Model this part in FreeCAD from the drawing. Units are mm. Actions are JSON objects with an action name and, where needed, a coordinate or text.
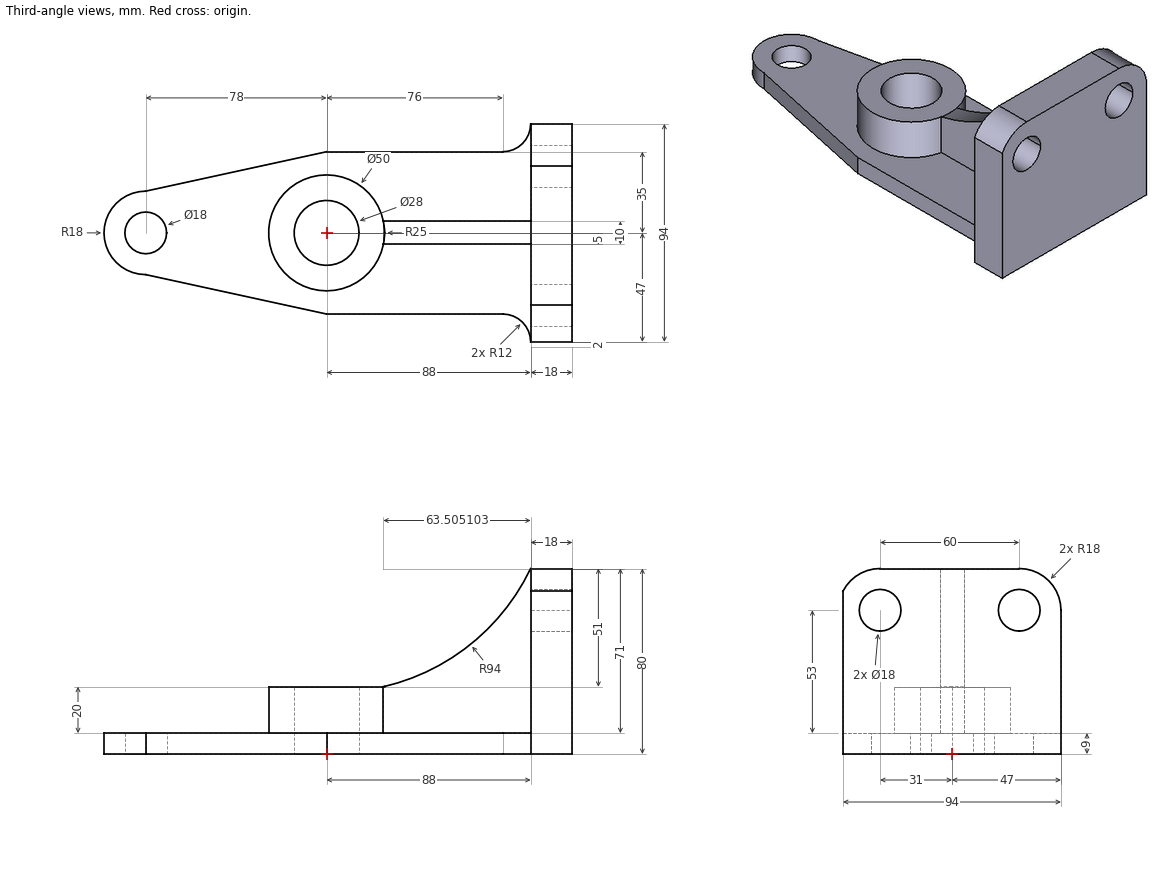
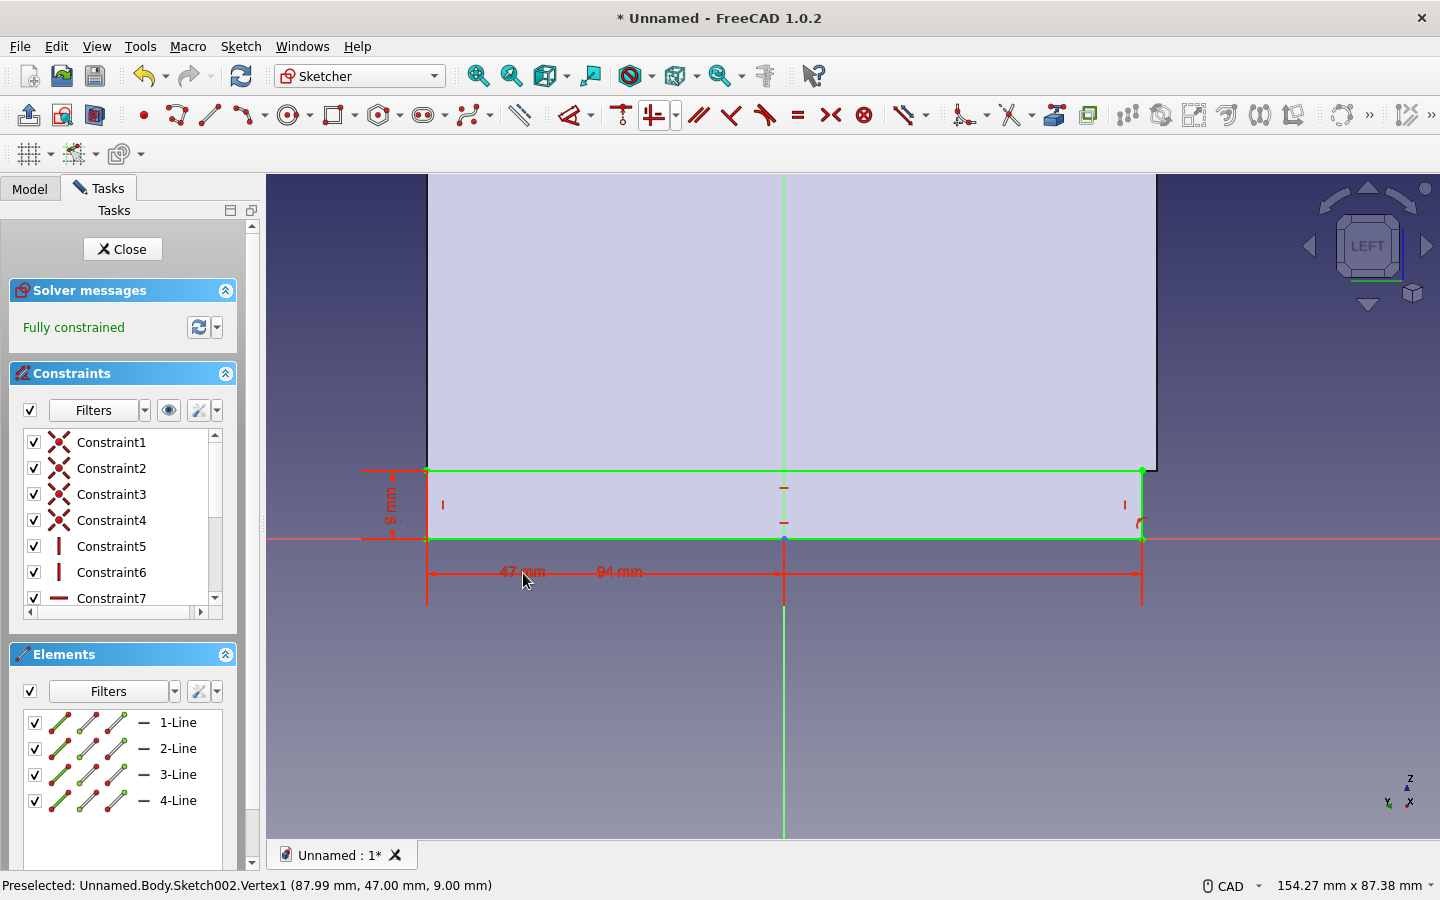
{"action": "left_click", "coordinate": [123, 249]}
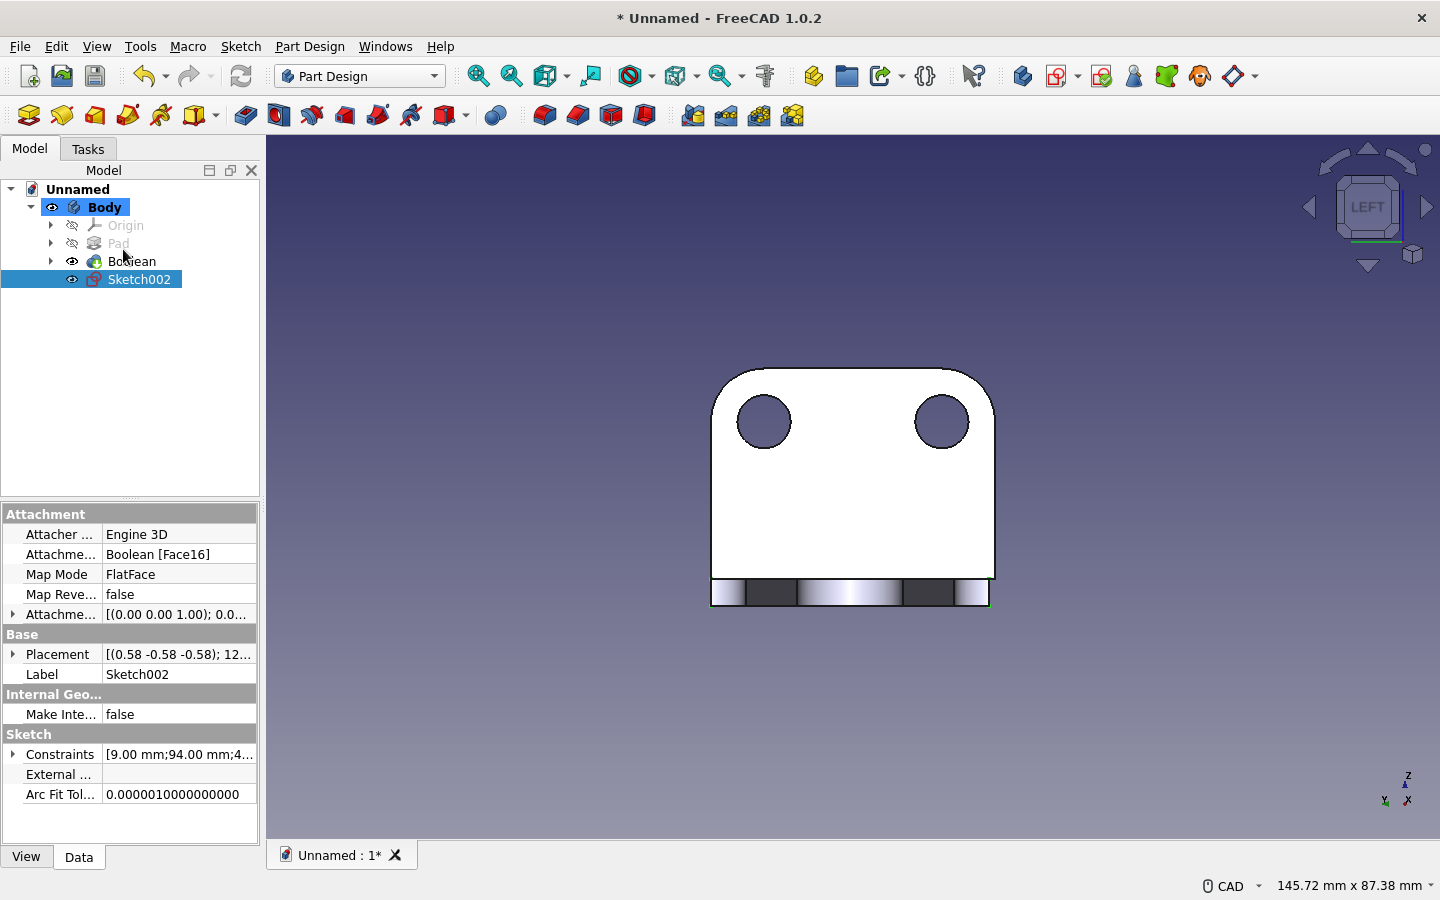
{"action": "left_click", "coordinate": [29, 116]}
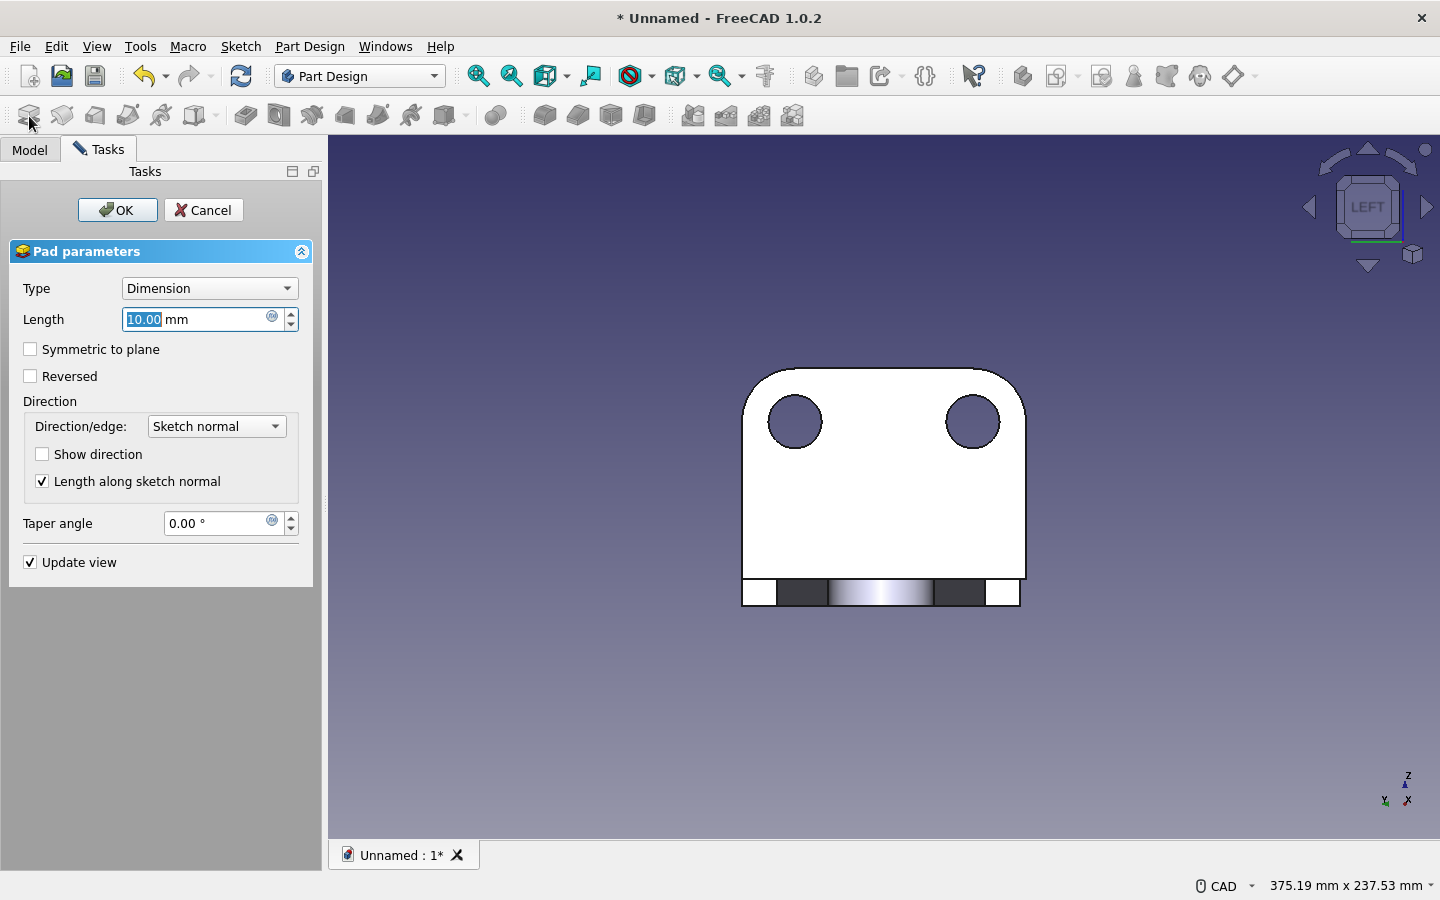
{"action": "type", "text": "18"}
{"action": "key", "text": "Tab"}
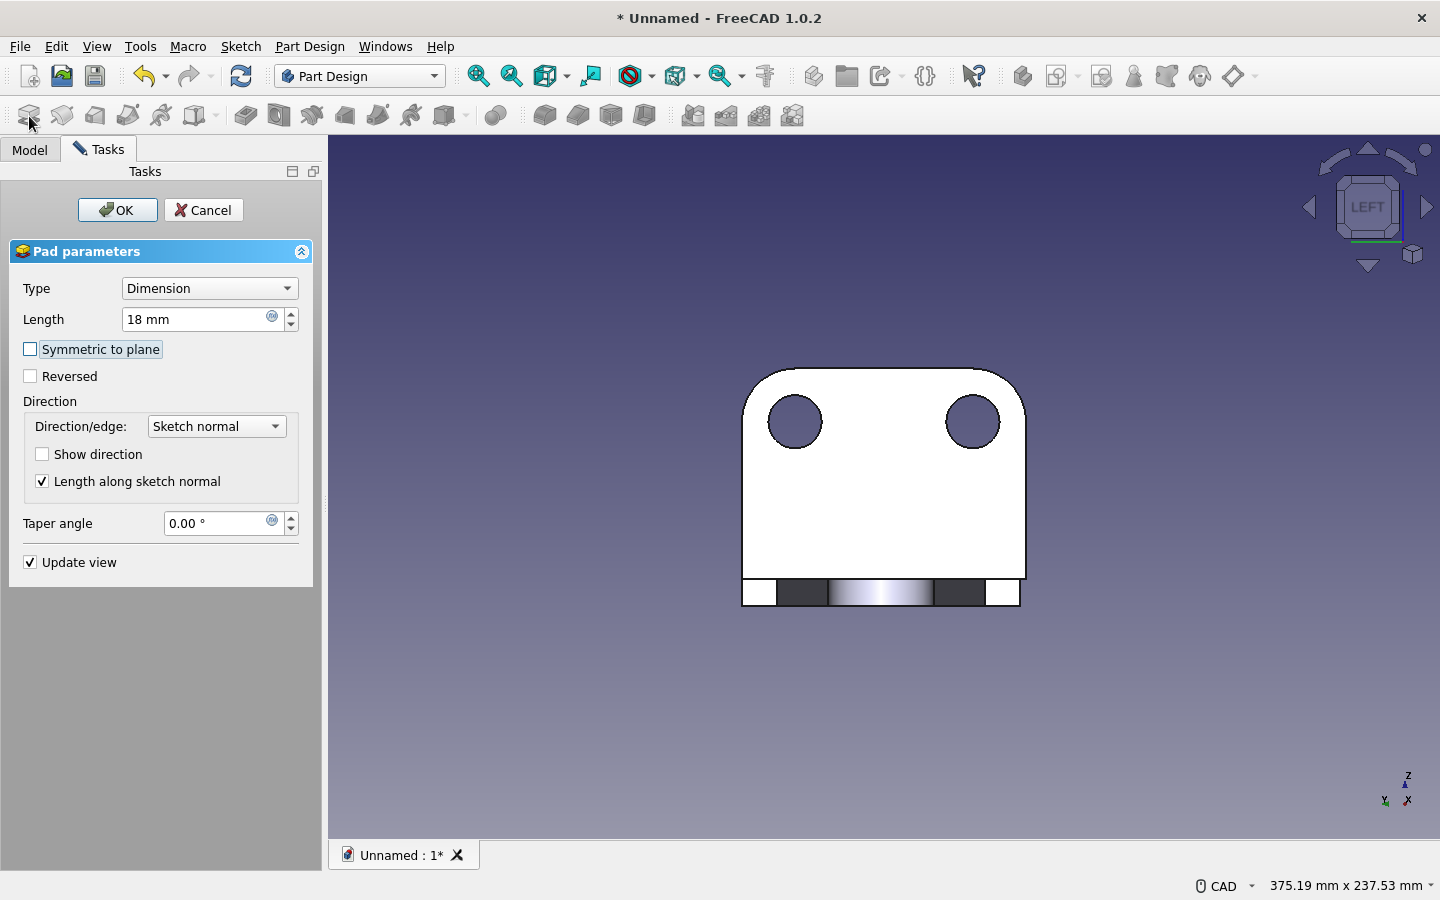
{"action": "left_click", "coordinate": [31, 376]}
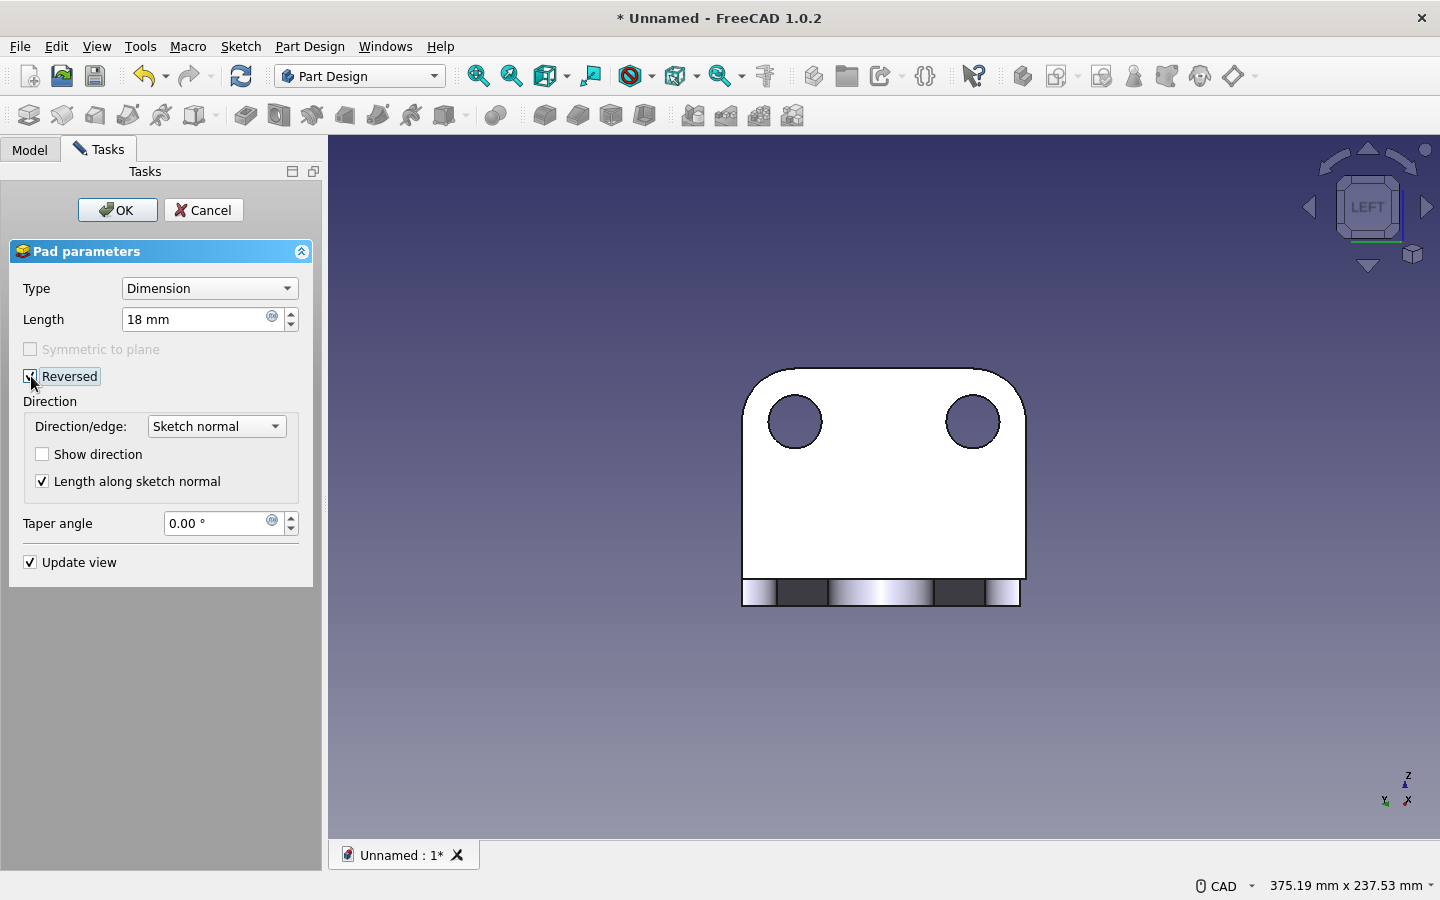
{"action": "left_click", "coordinate": [118, 210]}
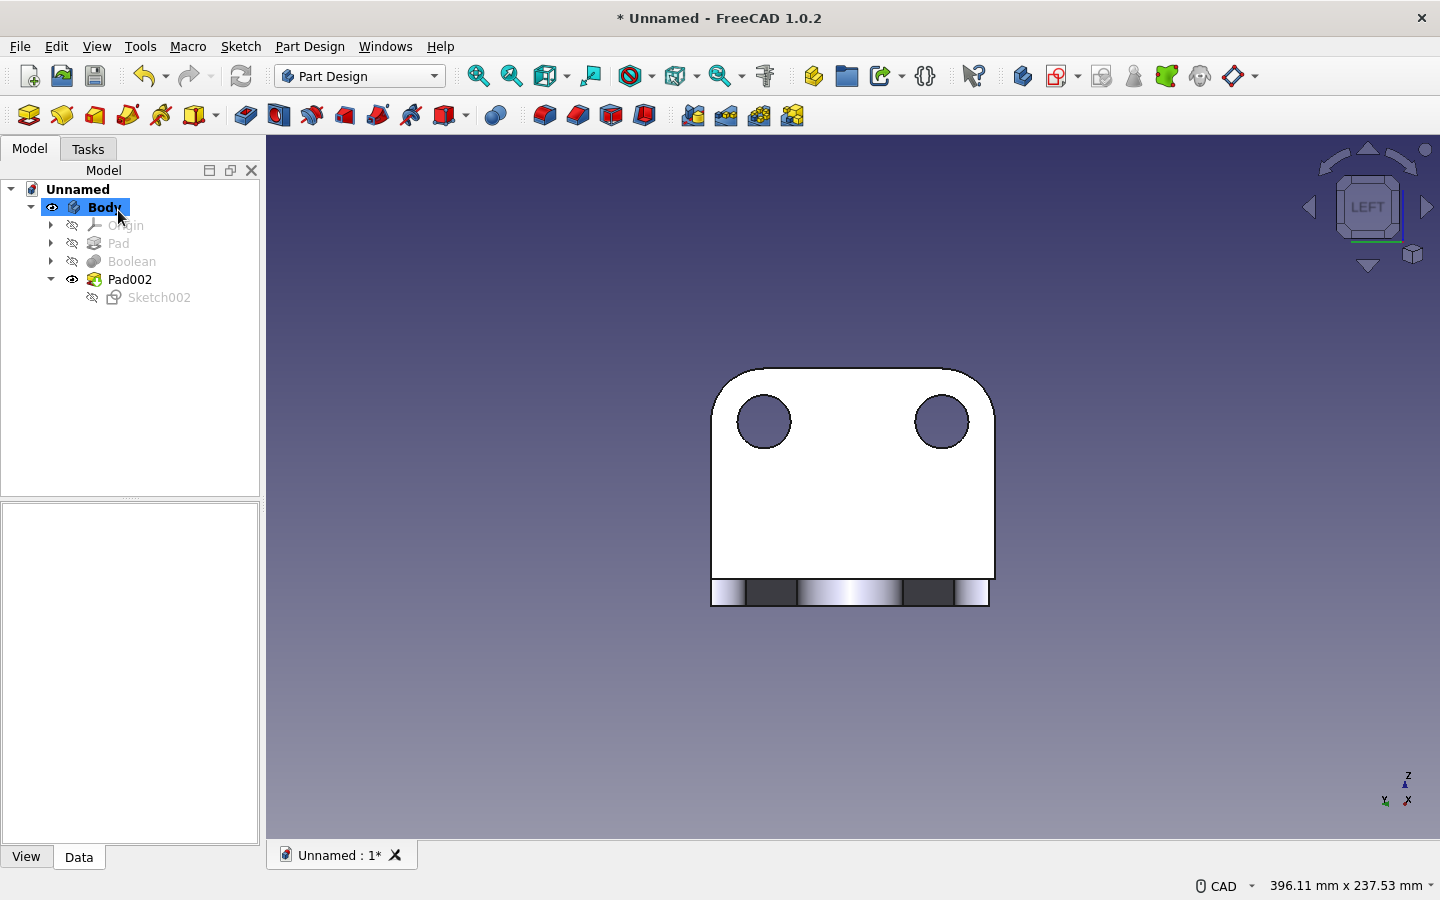
{"action": "left_click", "coordinate": [479, 76]}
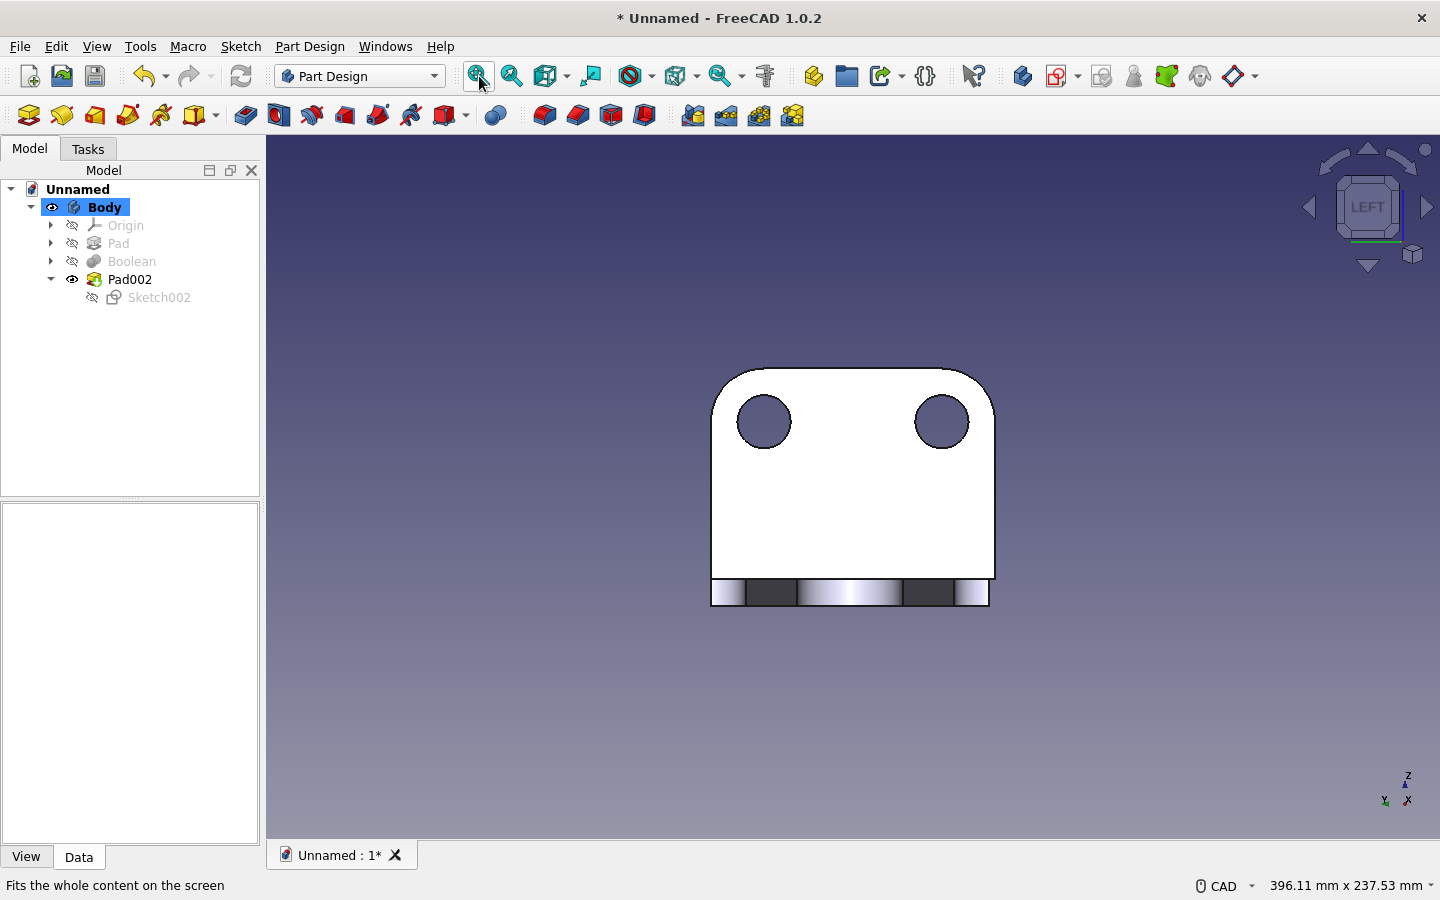
{"action": "key", "text": "0"}